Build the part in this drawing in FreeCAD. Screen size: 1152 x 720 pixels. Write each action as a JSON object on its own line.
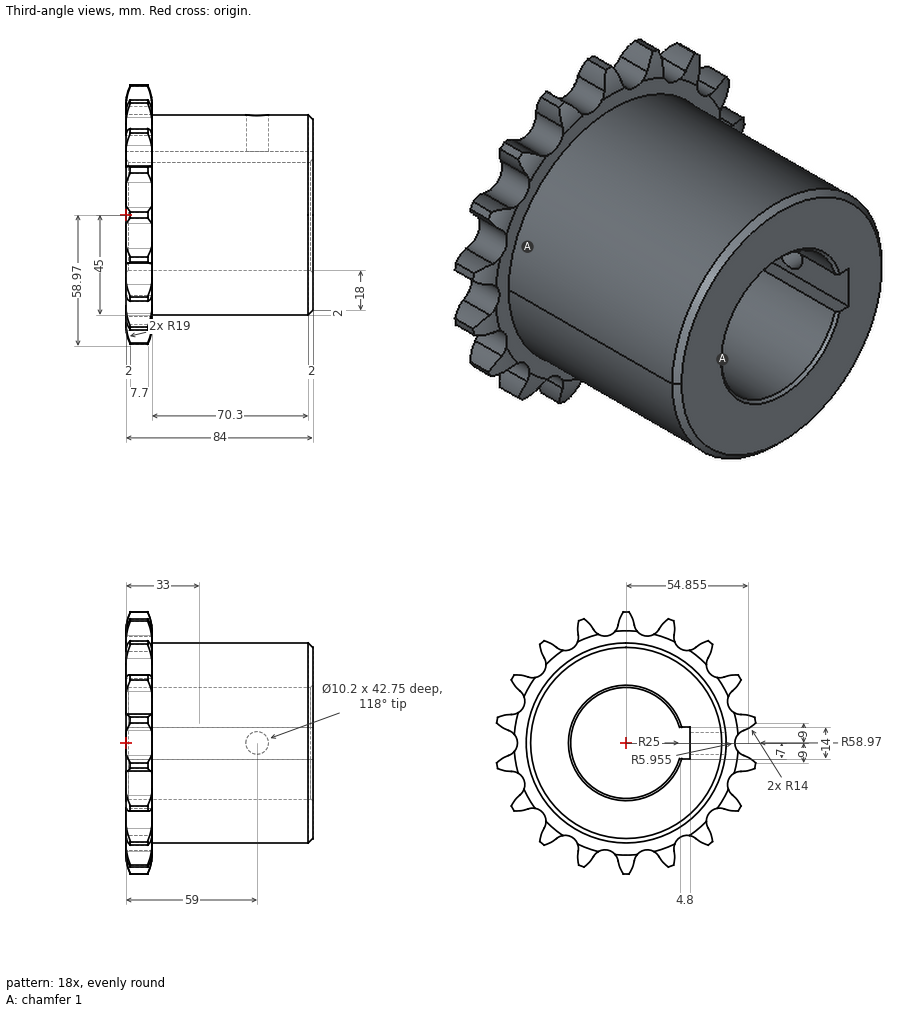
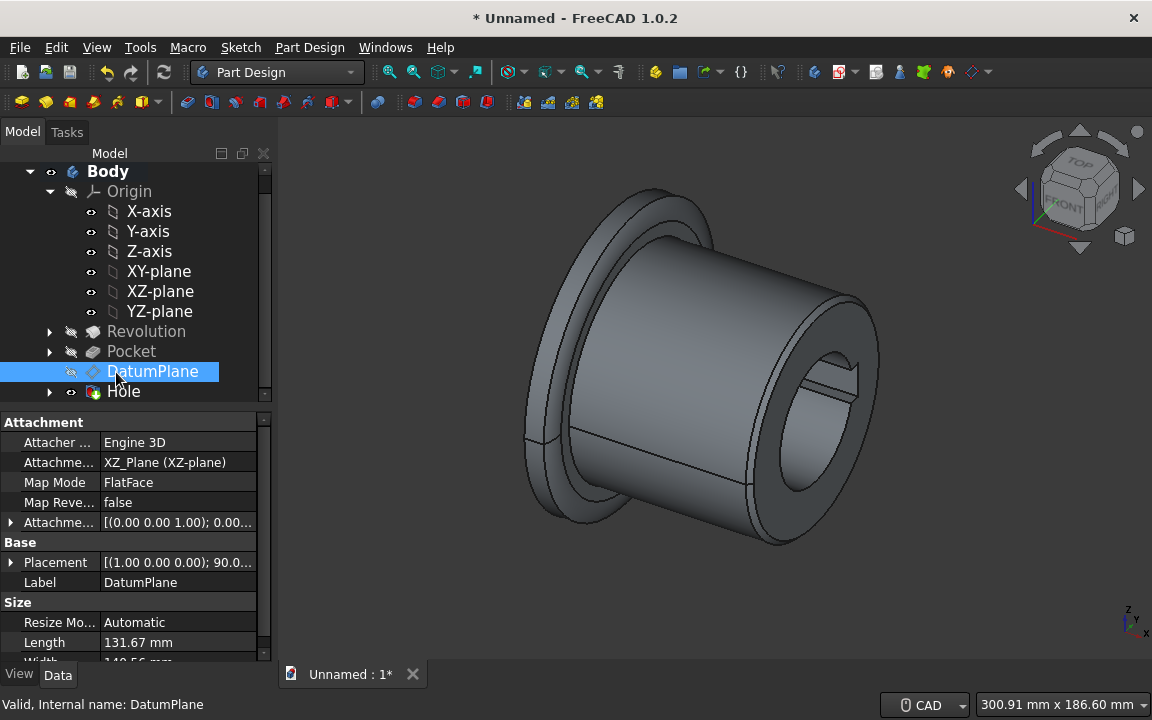
{"action": "left_click", "coordinate": [318, 619]}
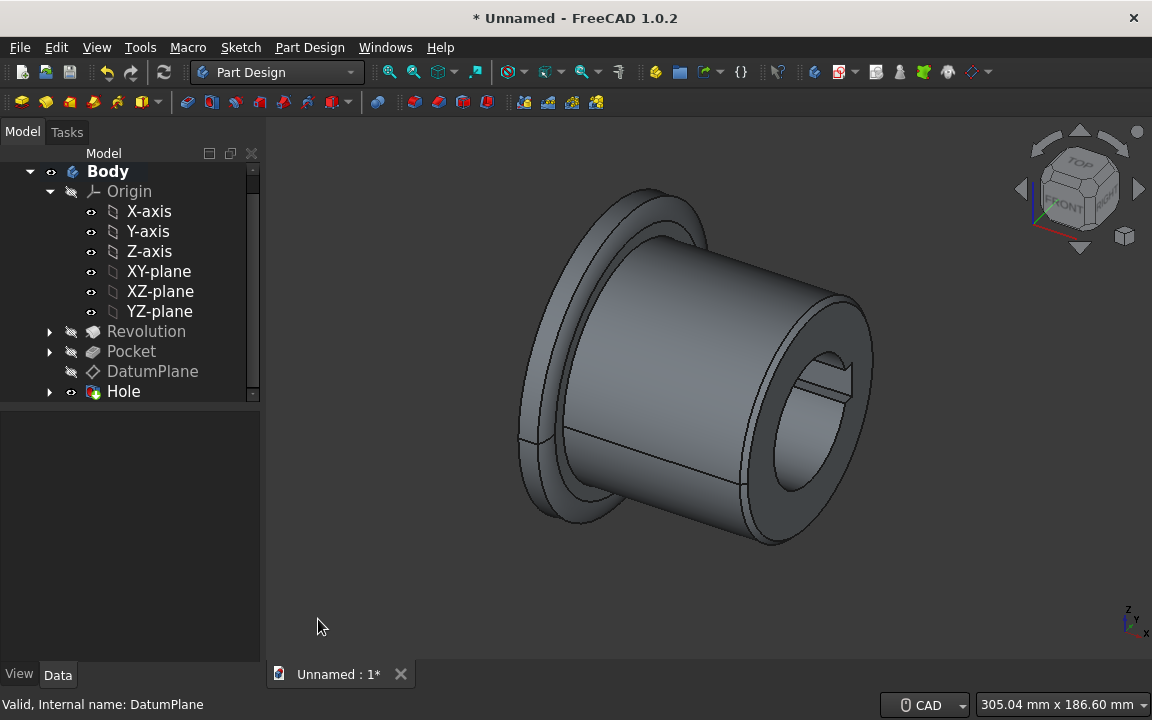
{"action": "left_click", "coordinate": [840, 72]}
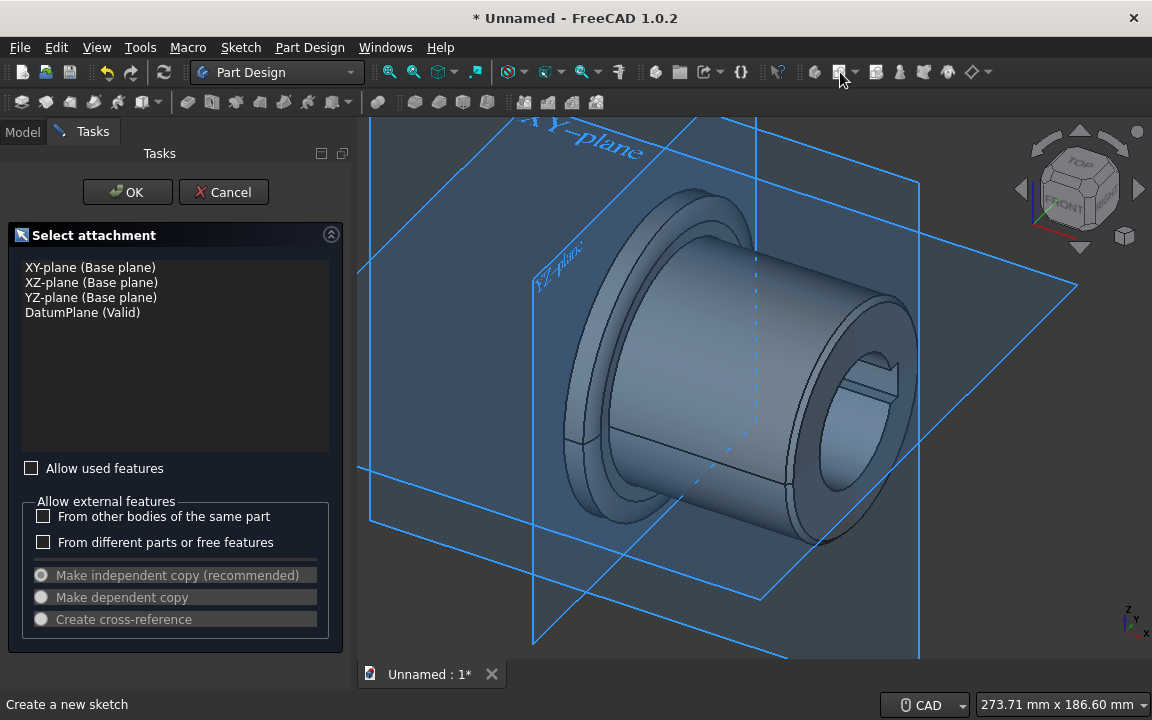
{"action": "left_click", "coordinate": [82, 298]}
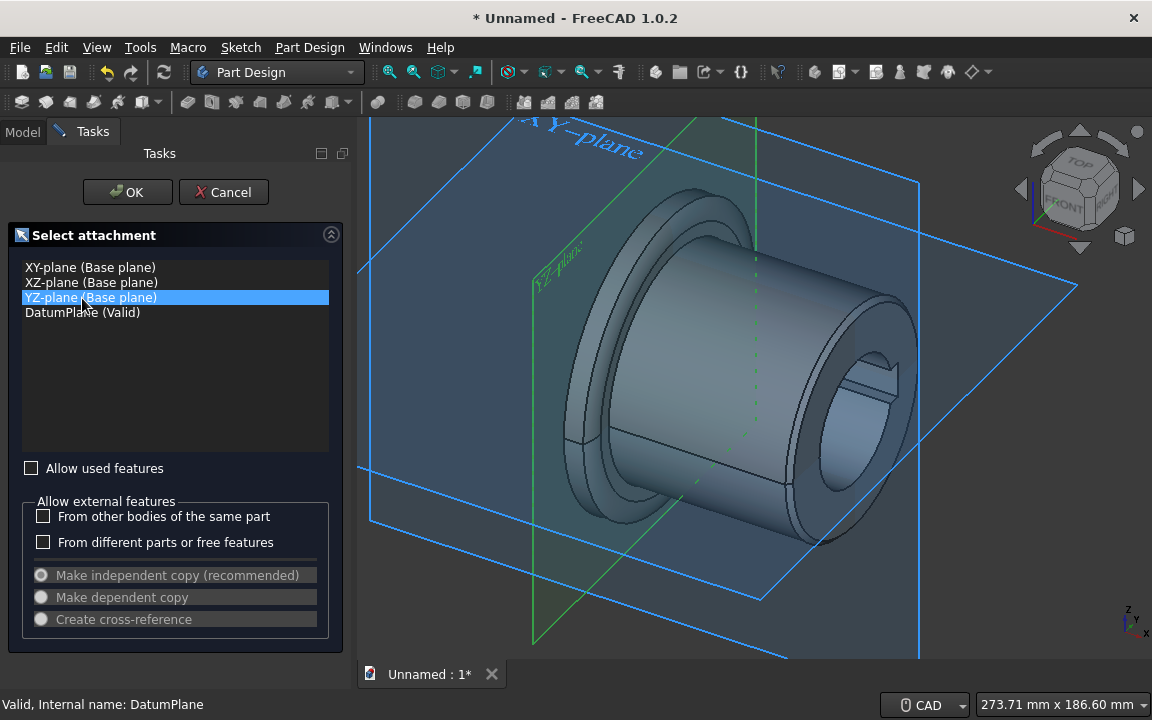
{"action": "left_click", "coordinate": [128, 192]}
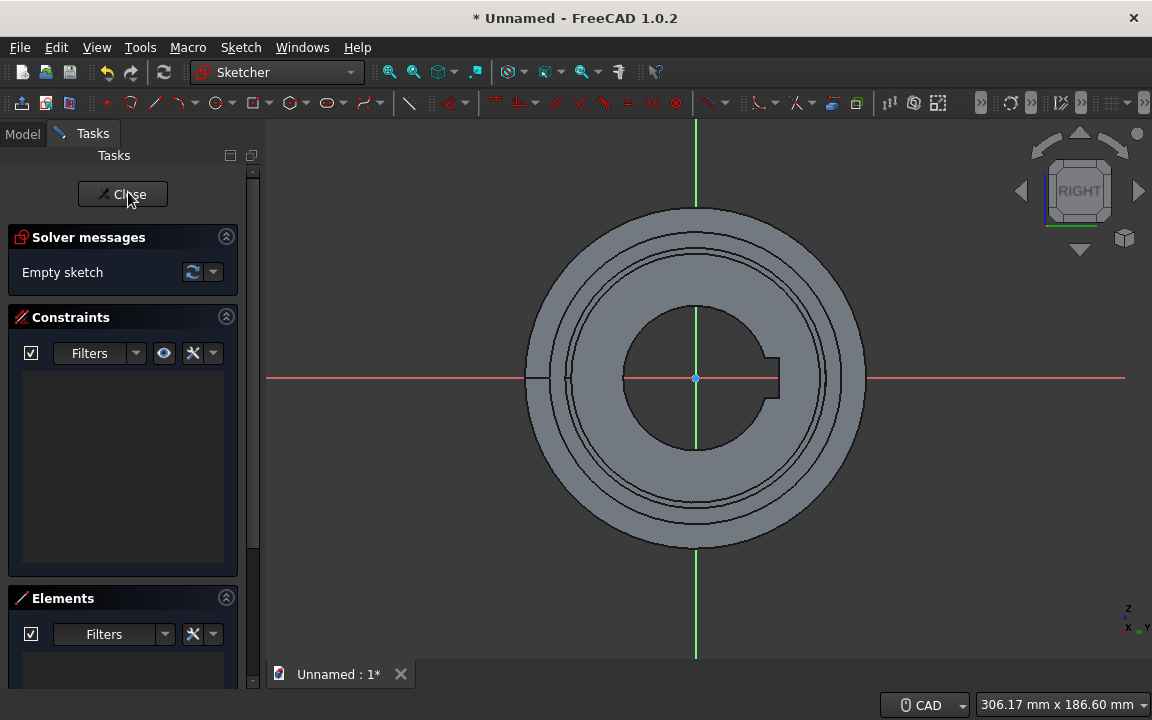
{"action": "key", "text": "q s"}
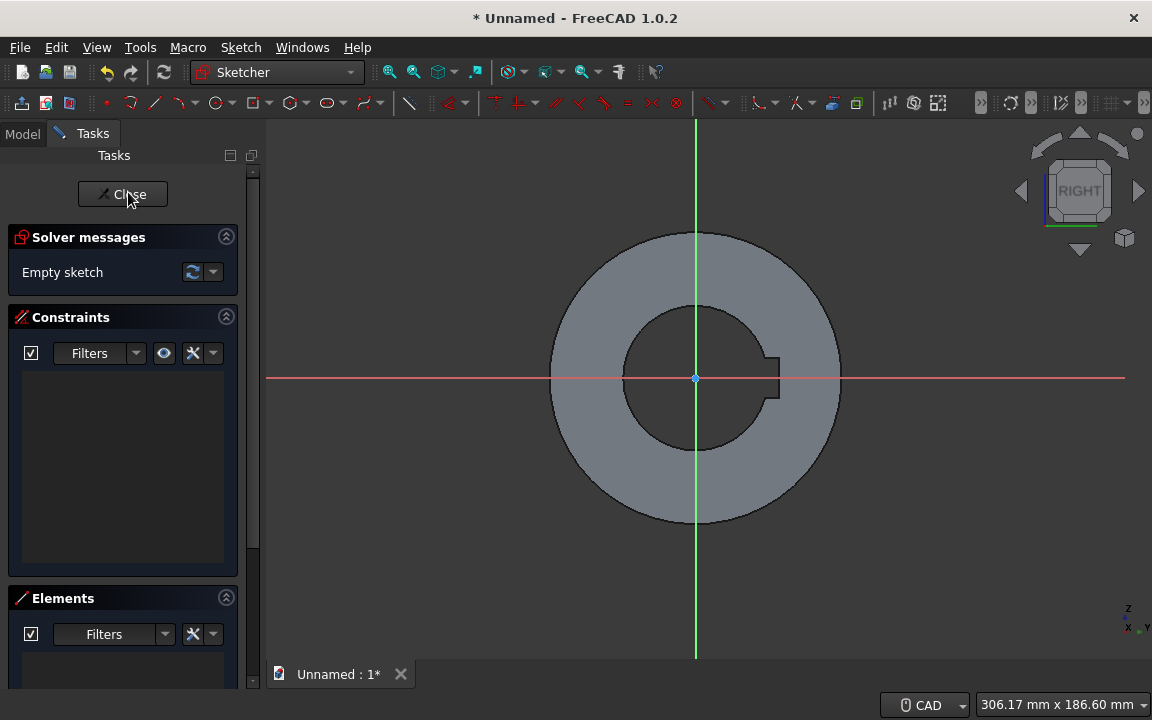
{"action": "scroll", "coordinate": [893, 376], "scroll_direction": "up", "scroll_amount": 9}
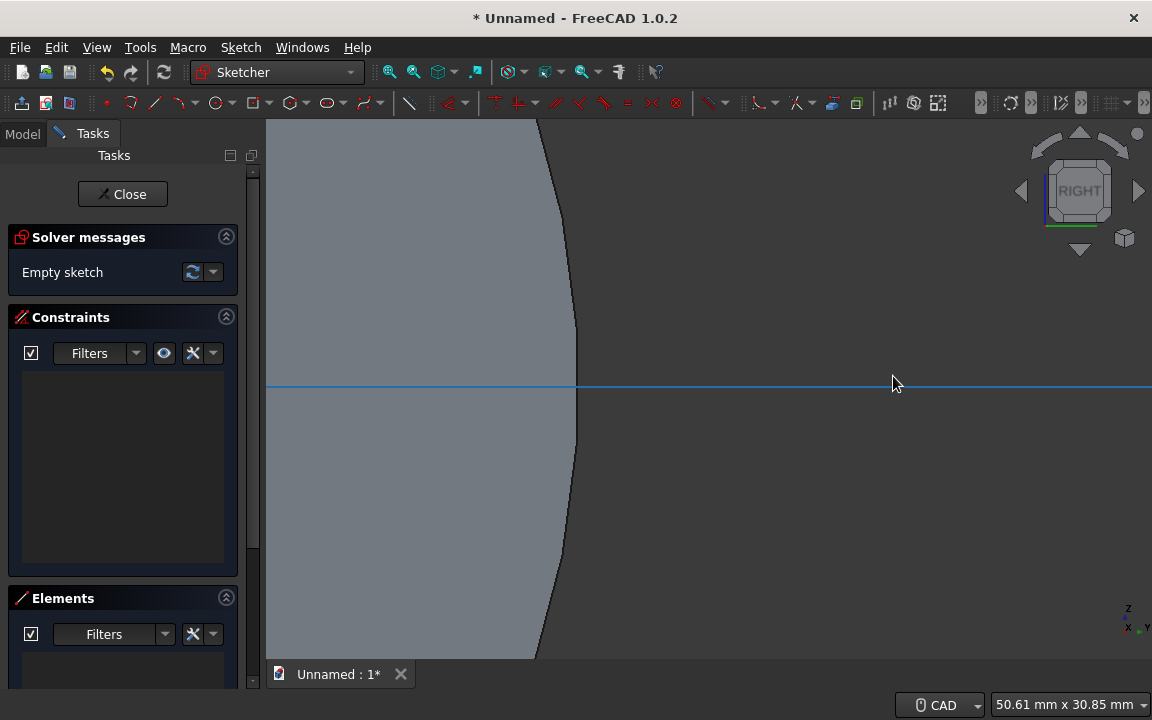
{"action": "left_click", "coordinate": [180, 104]}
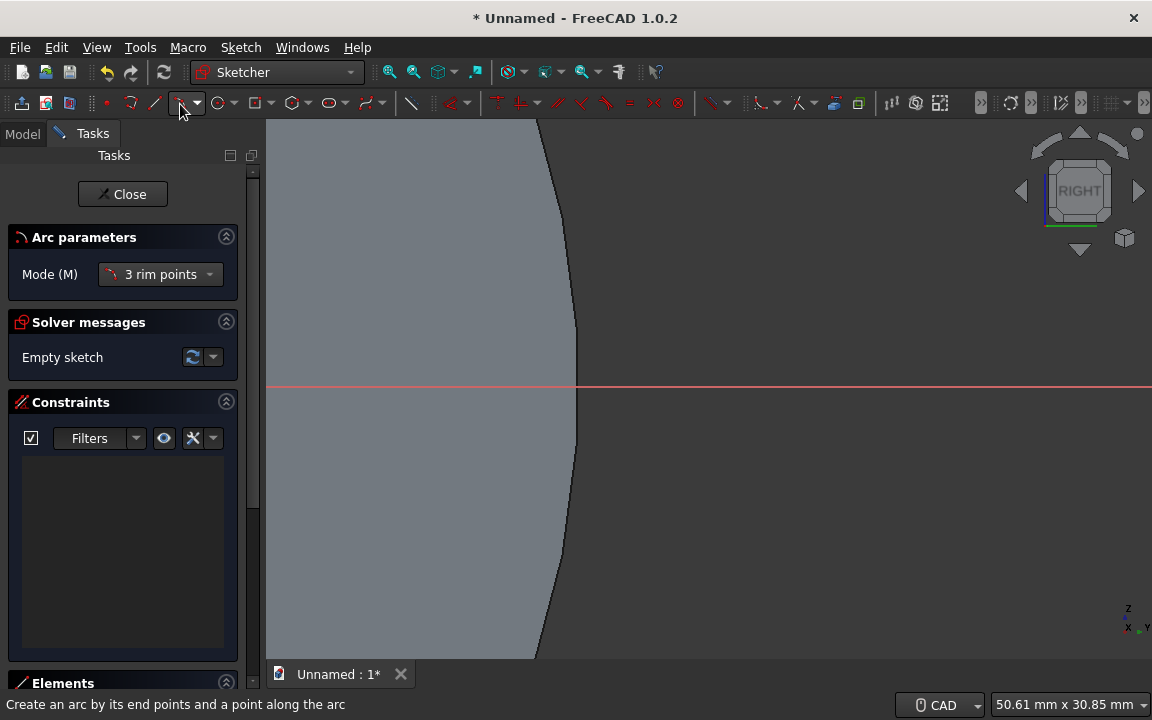
{"action": "left_click", "coordinate": [621, 485]}
{"action": "left_click", "coordinate": [621, 288]}
{"action": "left_click", "coordinate": [554, 361]}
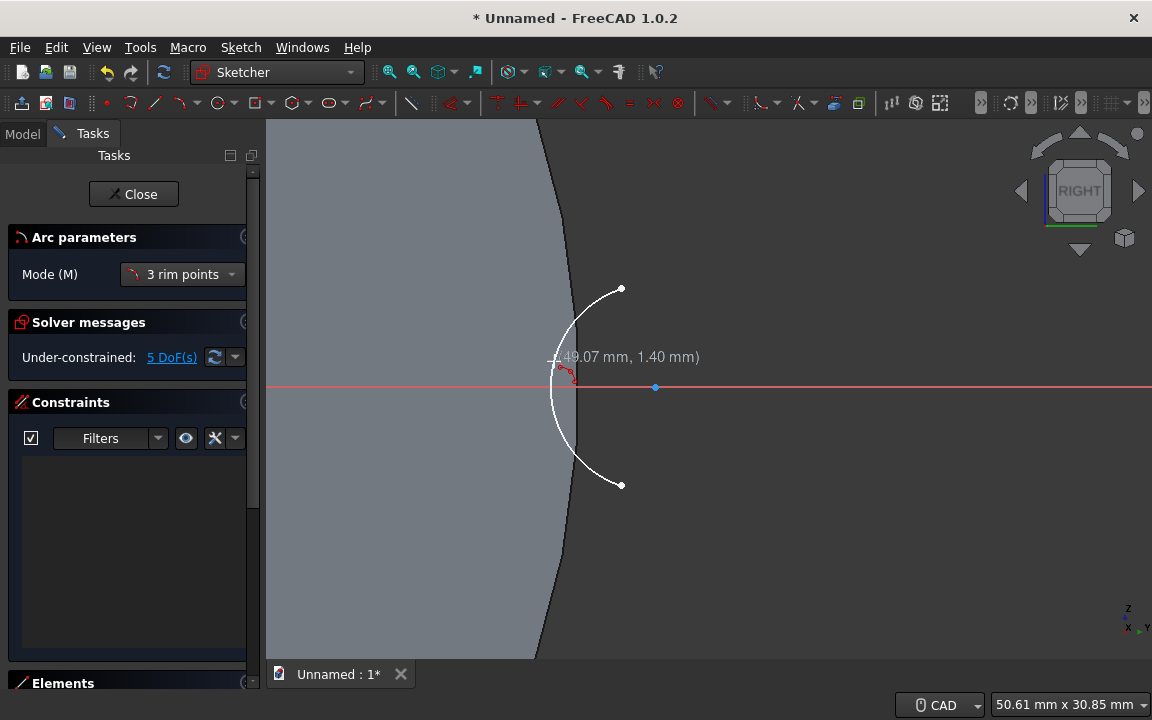
{"action": "left_click", "coordinate": [621, 289]}
{"action": "left_click", "coordinate": [715, 229]}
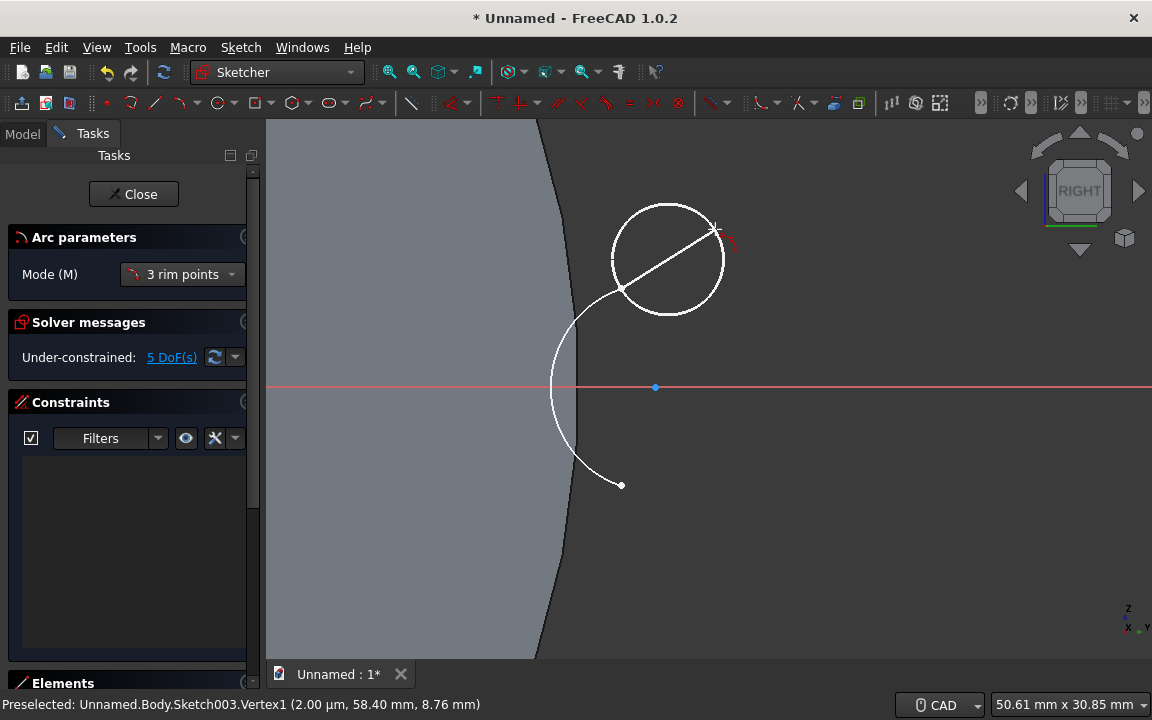
{"action": "scroll", "coordinate": [672, 264], "scroll_direction": "up", "scroll_amount": 5}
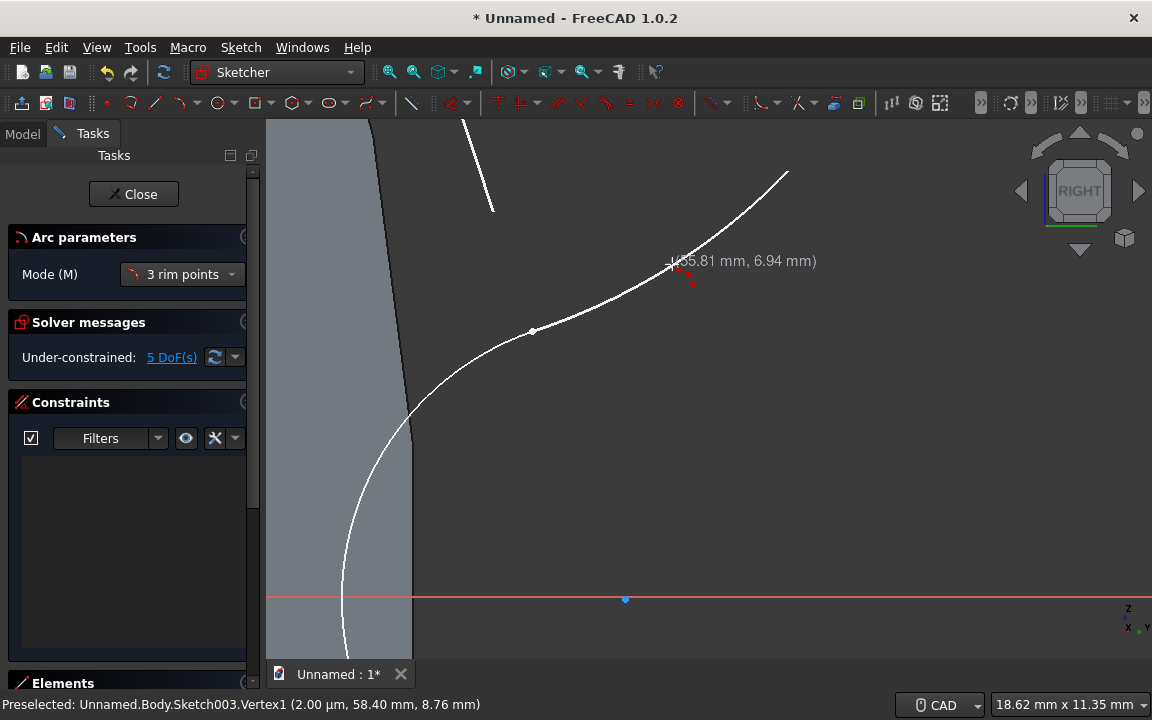
{"action": "left_click", "coordinate": [670, 263]}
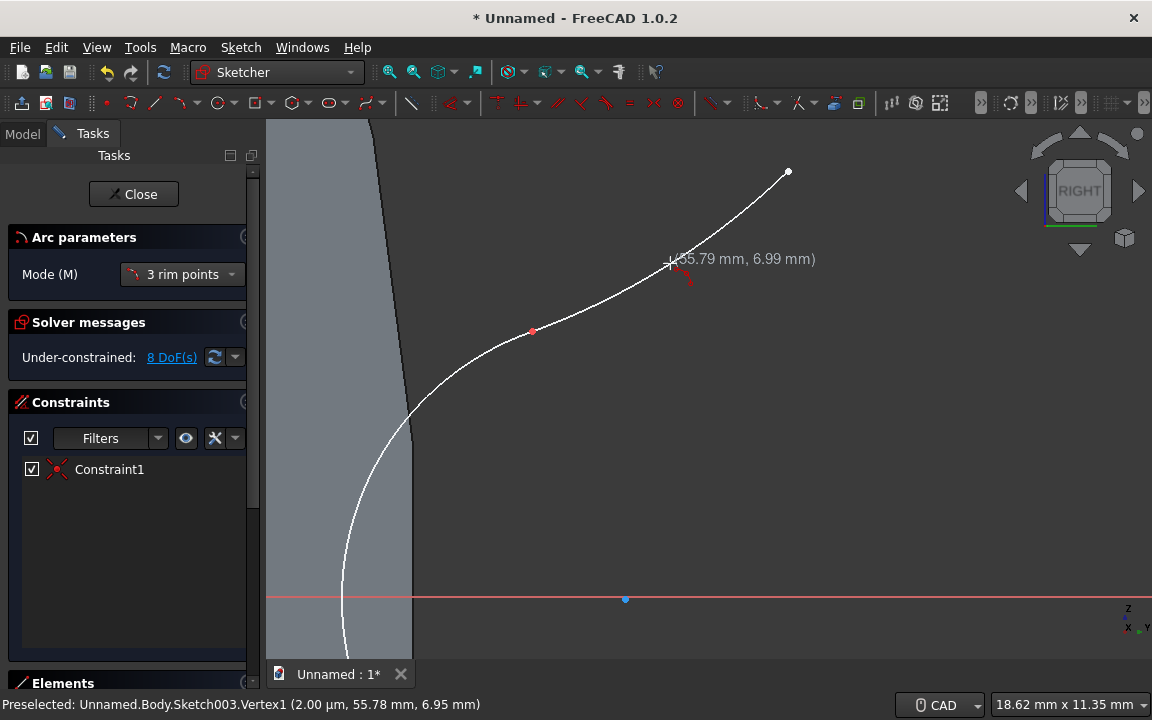
{"action": "left_click", "coordinate": [788, 171]}